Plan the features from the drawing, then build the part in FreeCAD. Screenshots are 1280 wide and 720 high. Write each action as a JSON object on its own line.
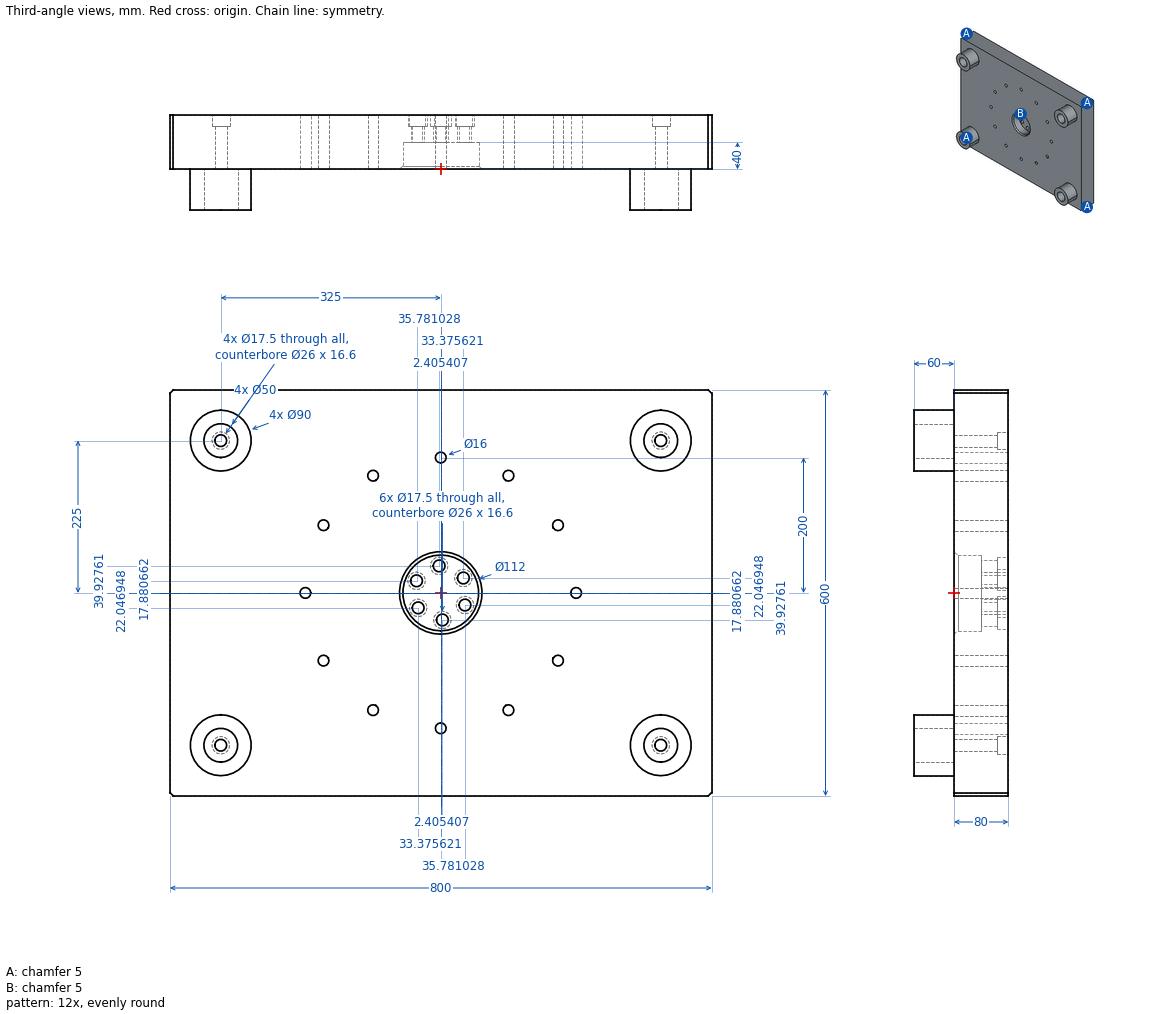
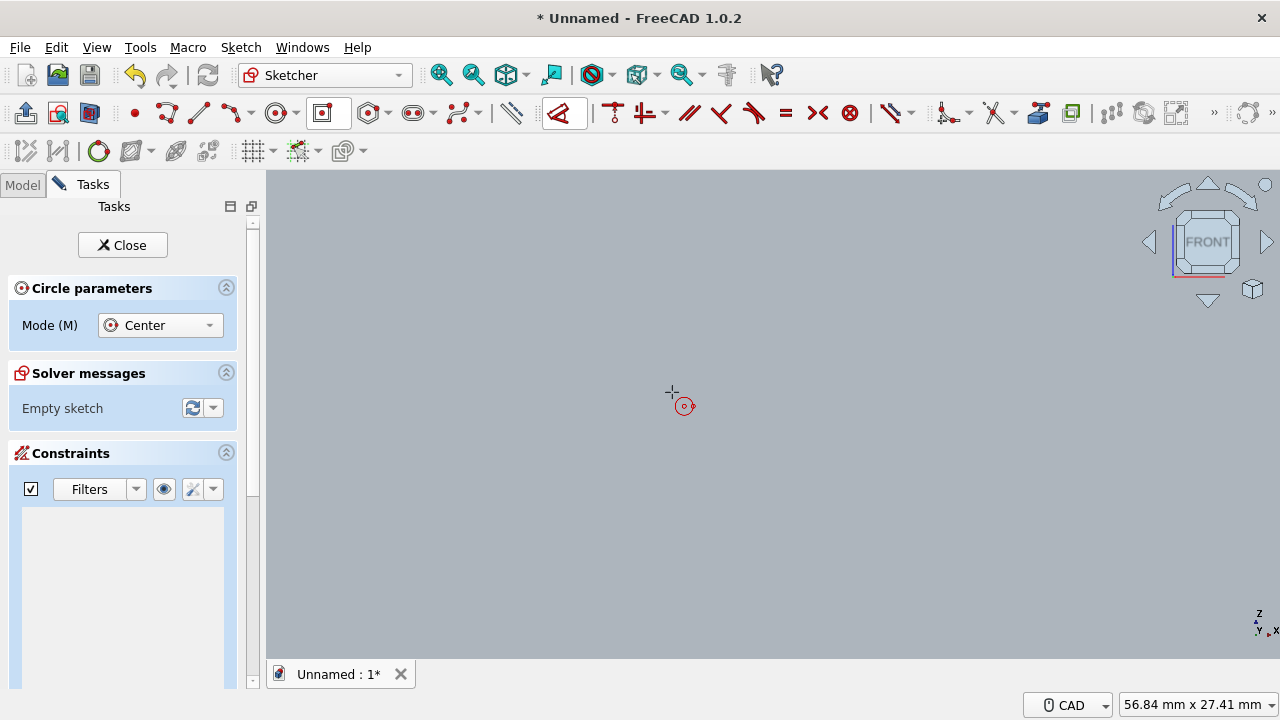
{"action": "left_click", "coordinate": [704, 414]}
{"action": "mouse_move", "coordinate": [805, 313]}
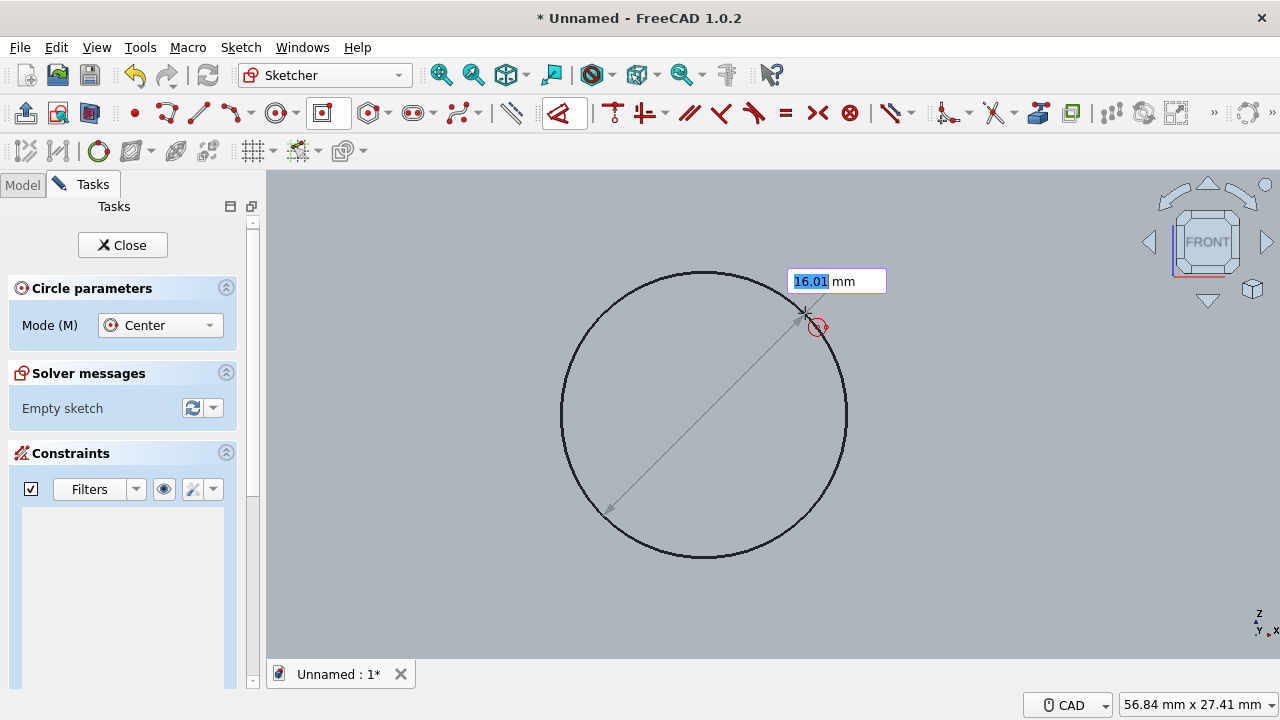
{"action": "type", "text": "16"}
{"action": "key", "text": "Return"}
{"action": "key", "text": "Escape"}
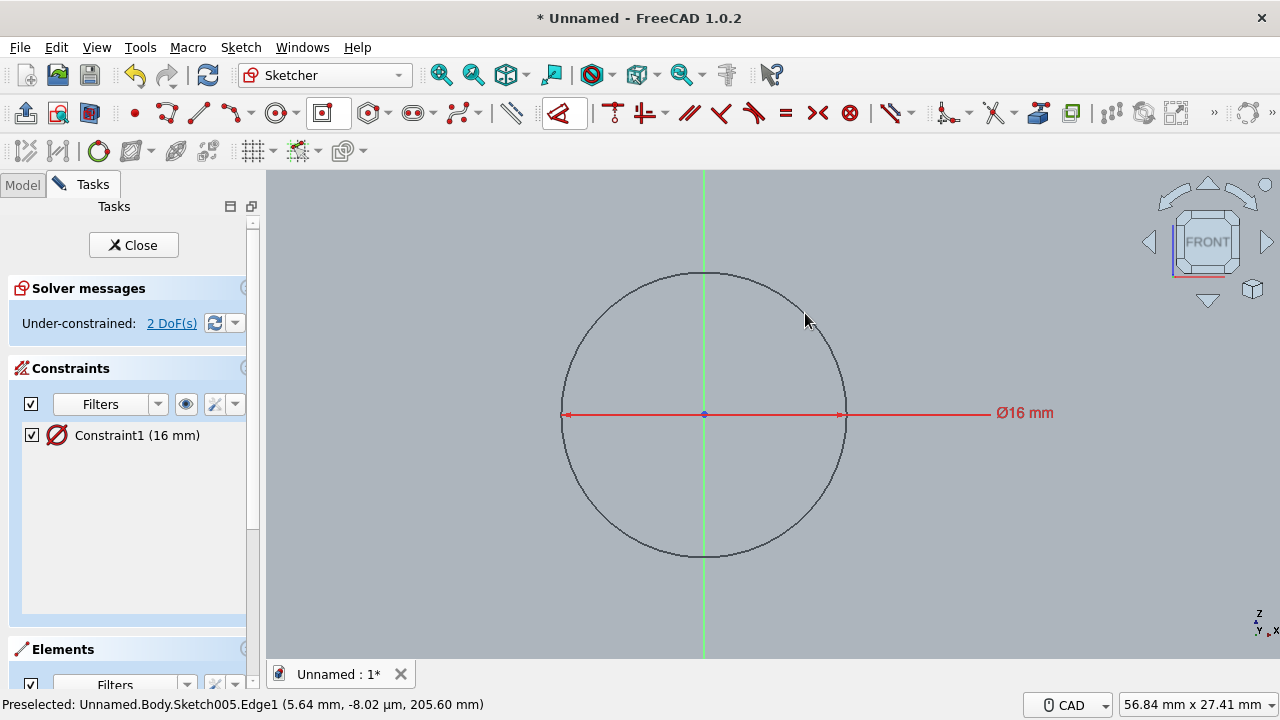
{"action": "left_click", "coordinate": [704, 415]}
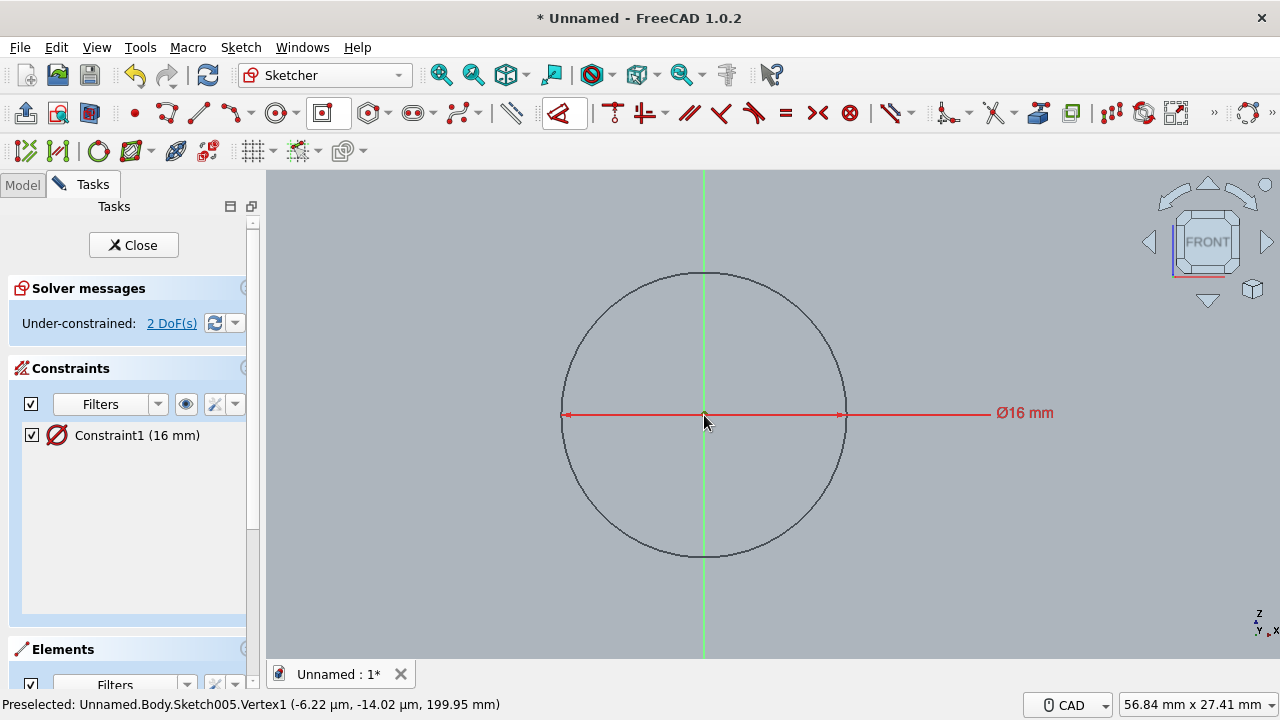
{"action": "left_click", "coordinate": [704, 600]}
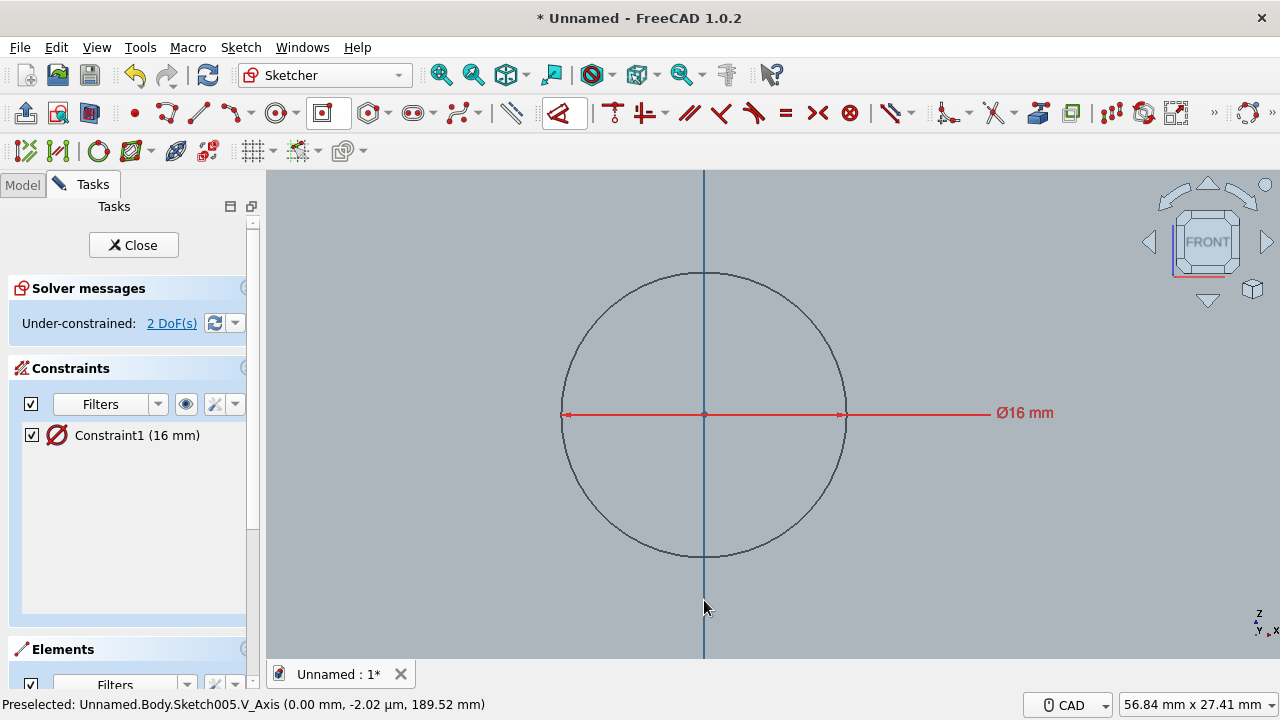
{"action": "key", "text": "c"}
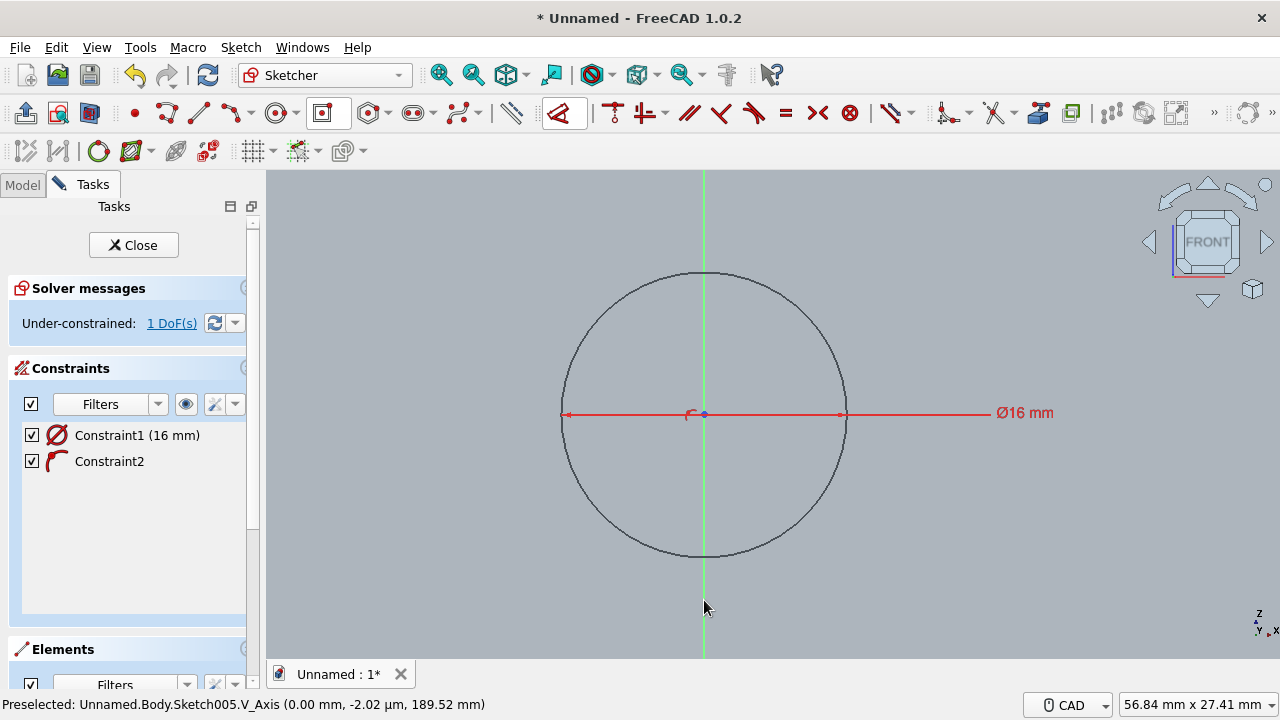
{"action": "left_click", "coordinate": [704, 415]}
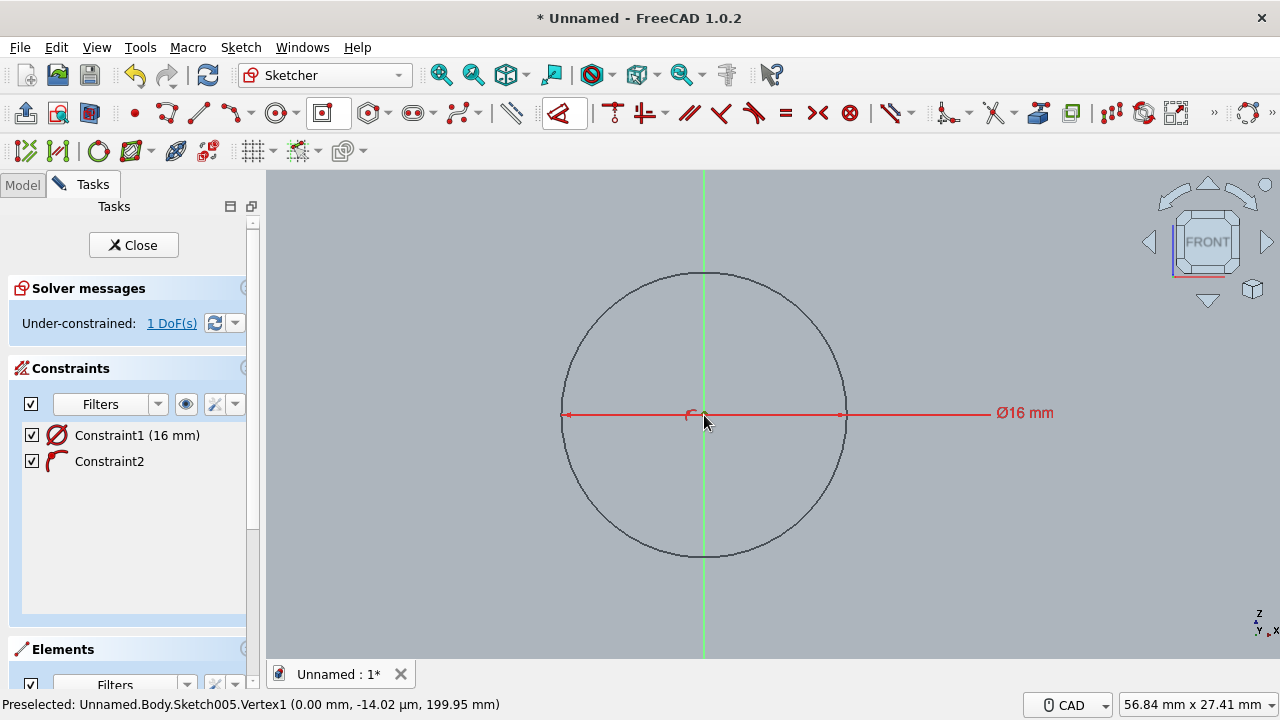
{"action": "key", "text": "i"}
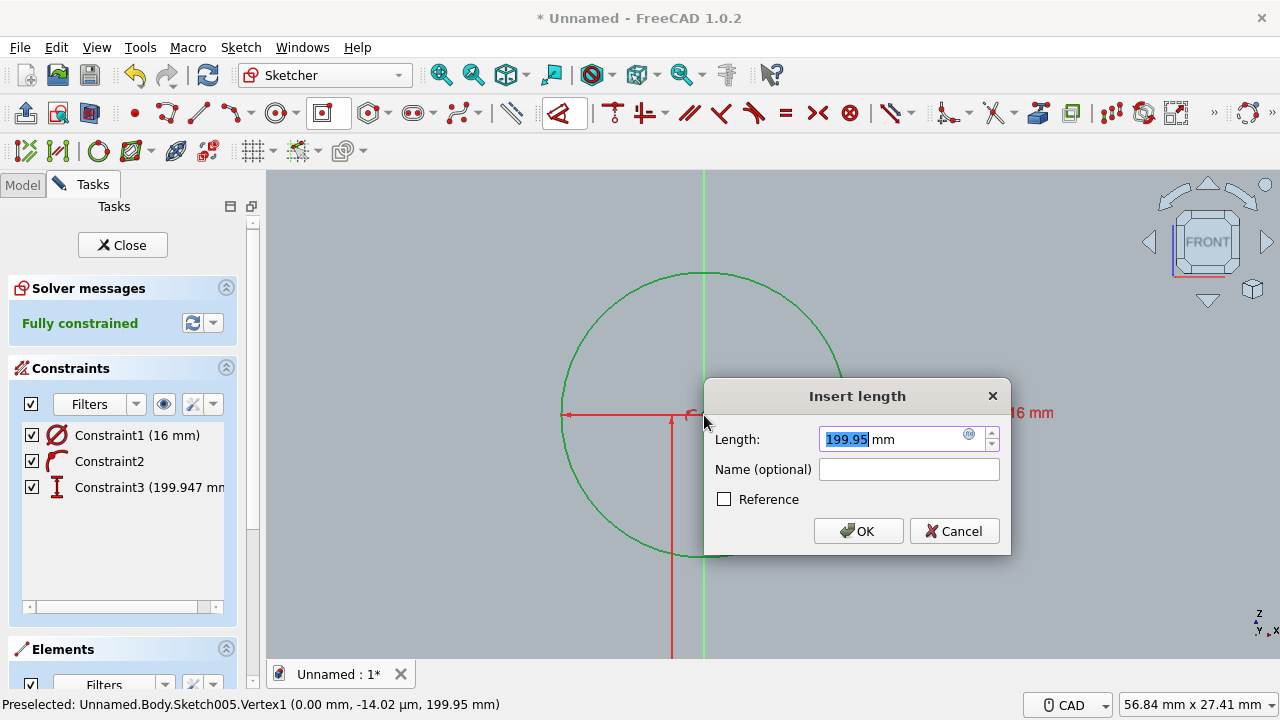
{"action": "type", "text": "200"}
{"action": "key", "text": "Return"}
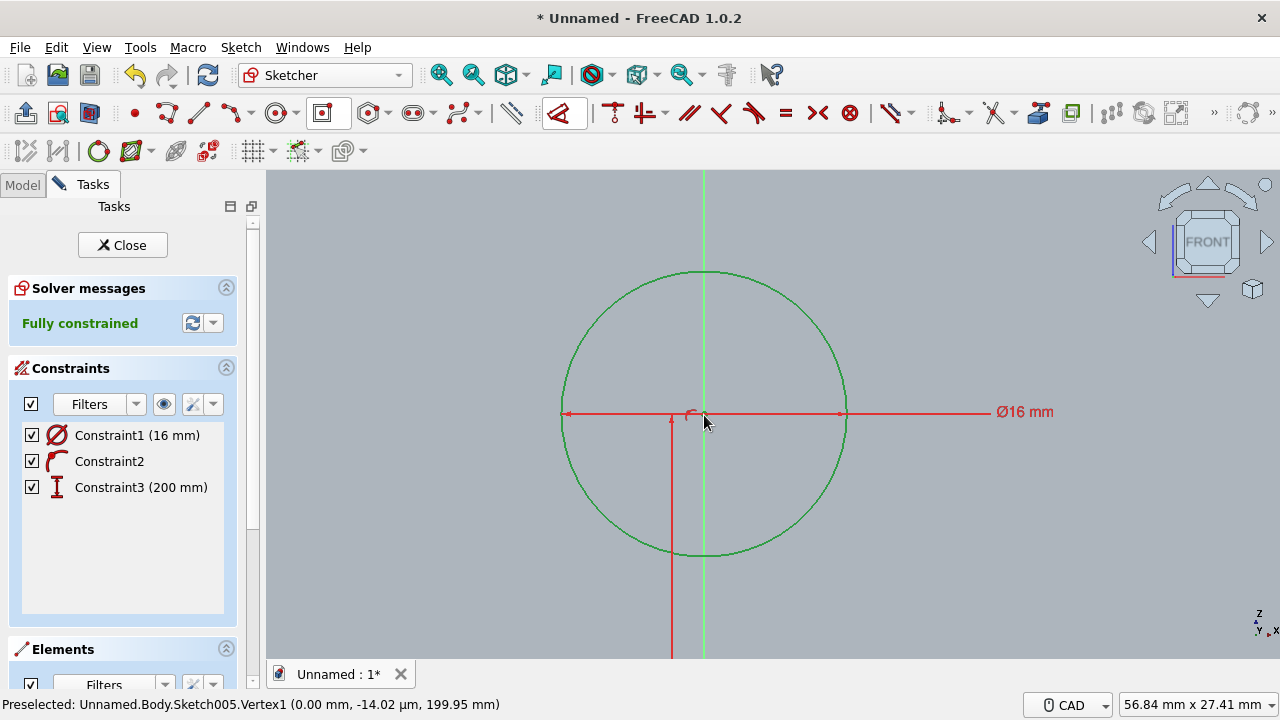
{"action": "left_click", "coordinate": [123, 245]}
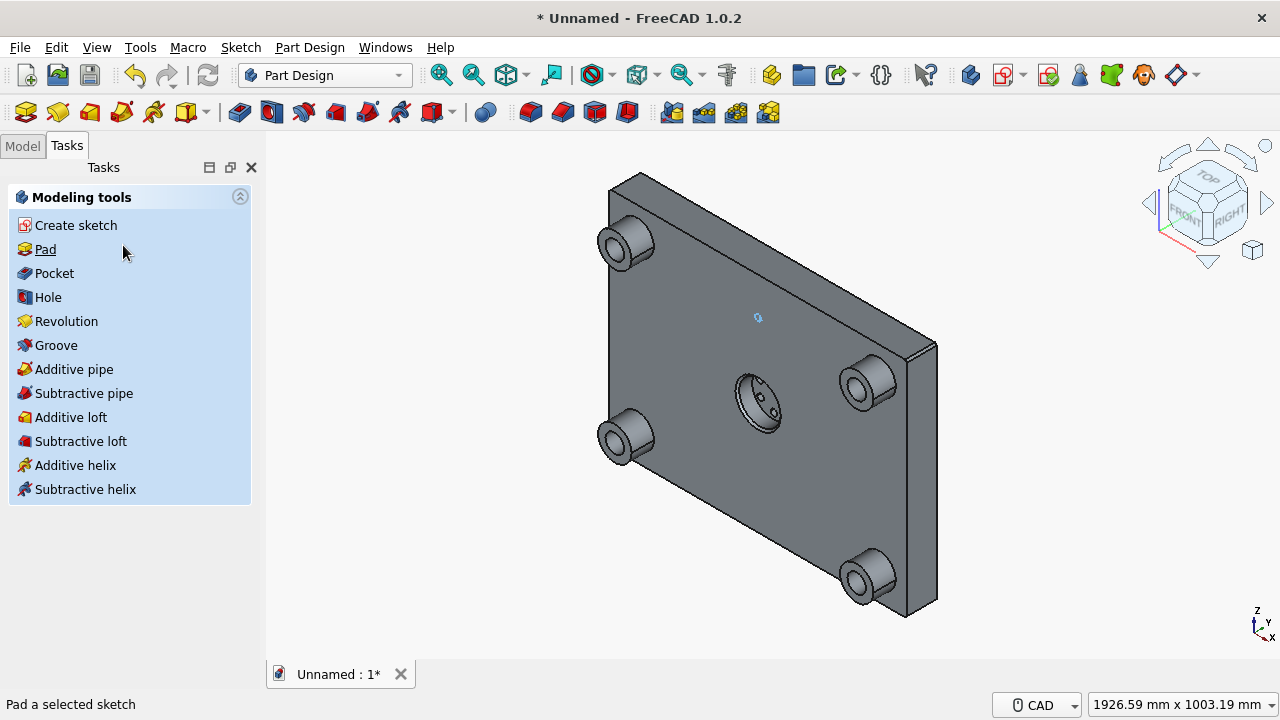
{"action": "left_click", "coordinate": [240, 112]}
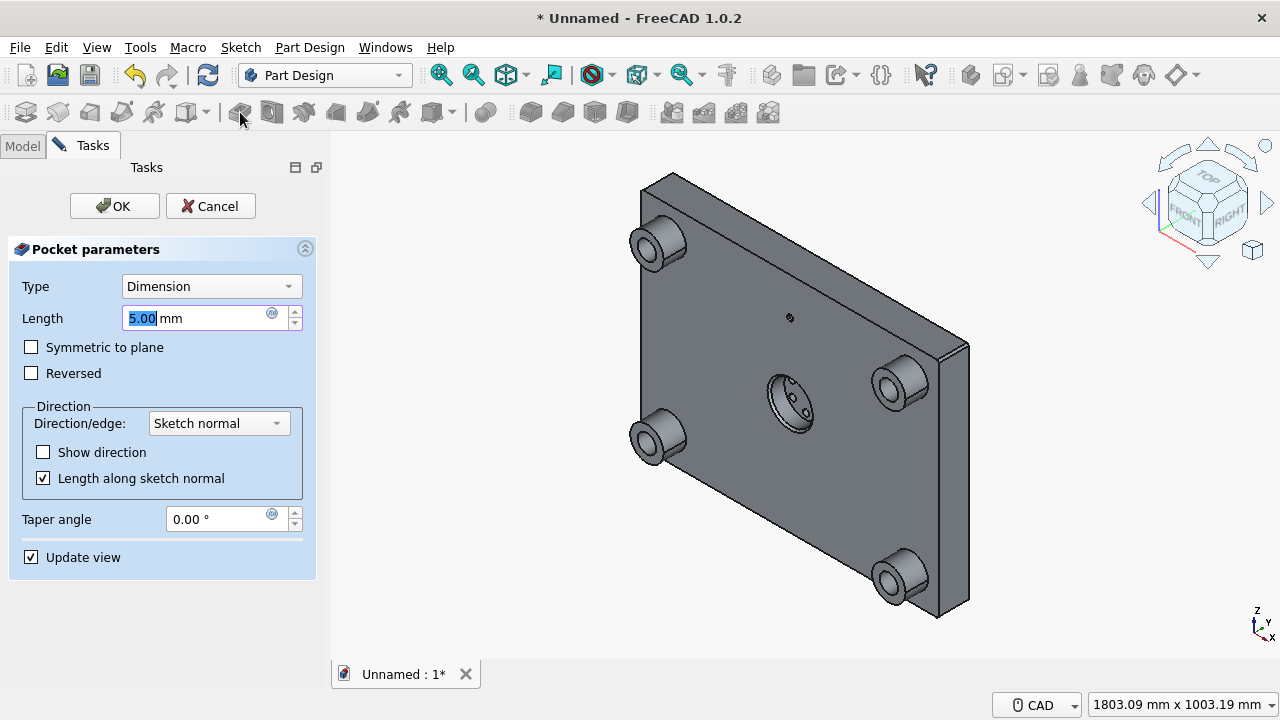
{"action": "left_click", "coordinate": [212, 286]}